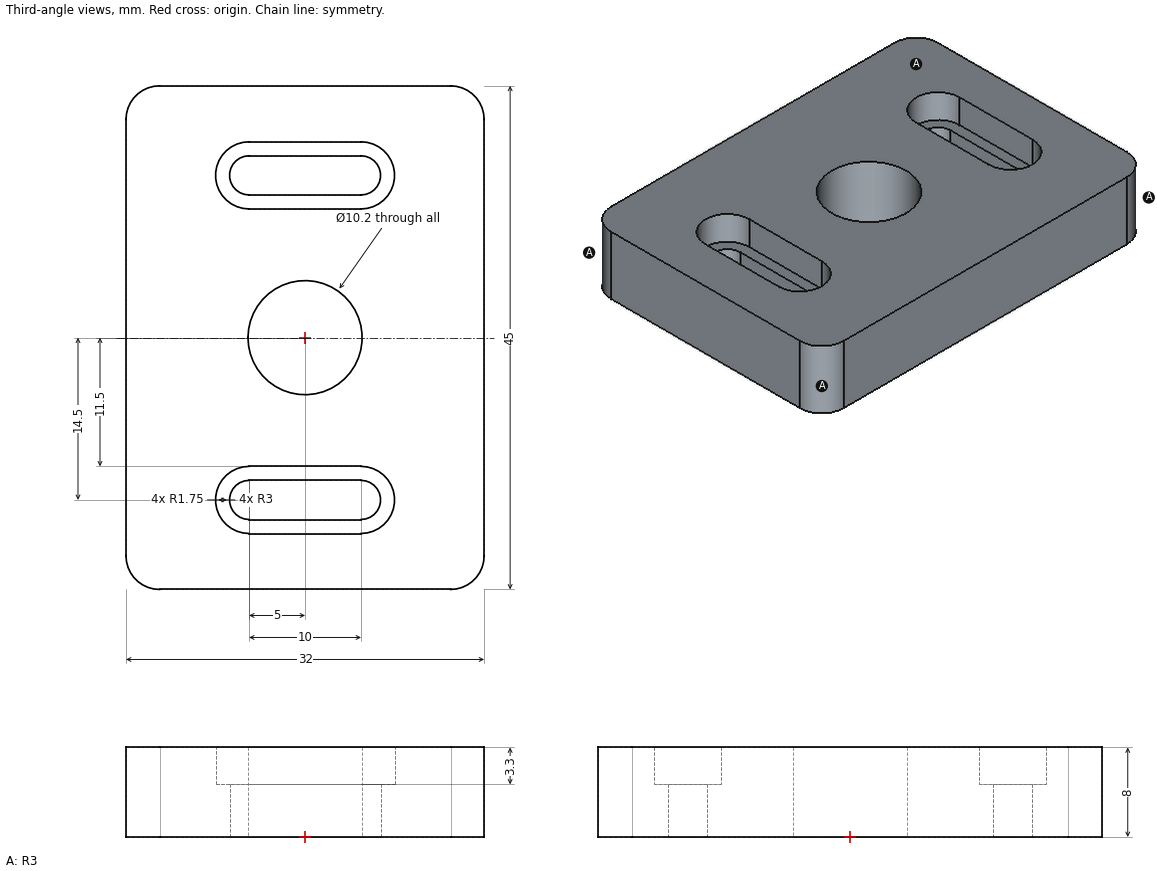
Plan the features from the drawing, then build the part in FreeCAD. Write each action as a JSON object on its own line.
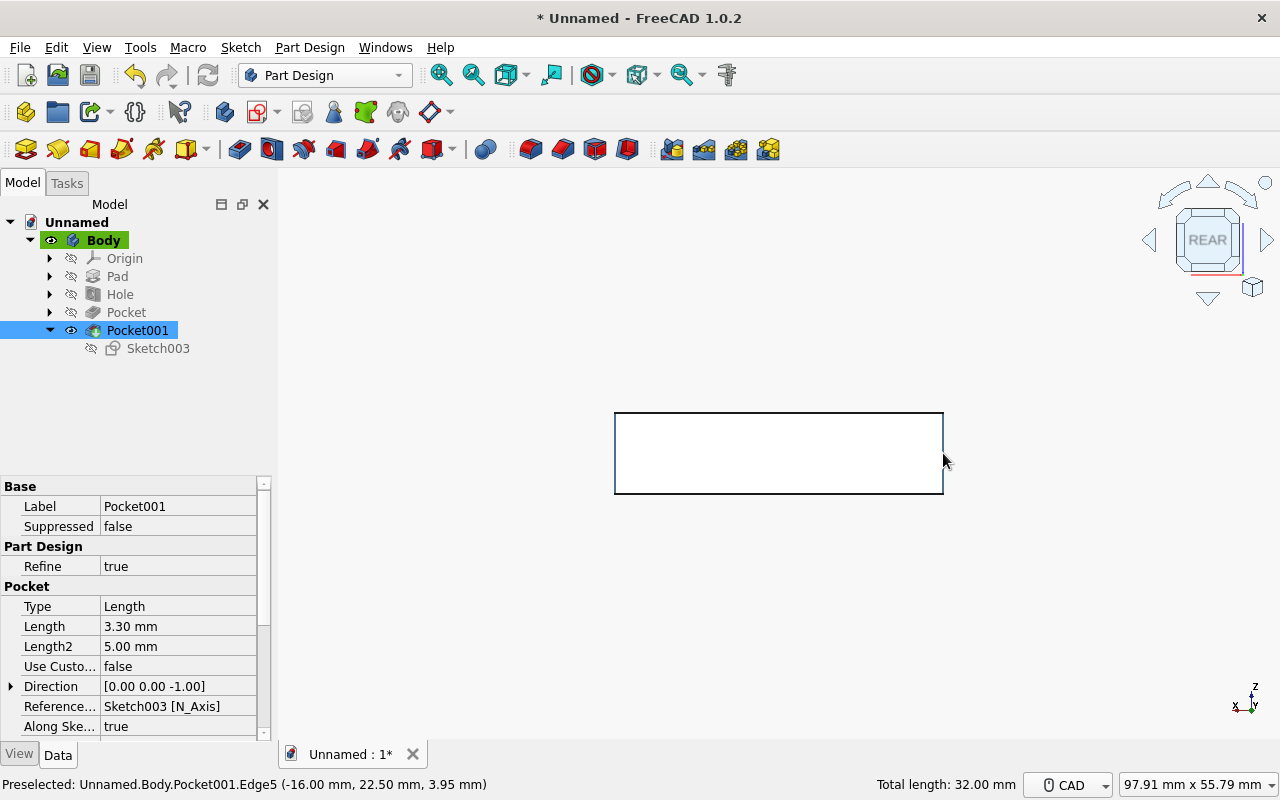
{"action": "left_click", "coordinate": [532, 150]}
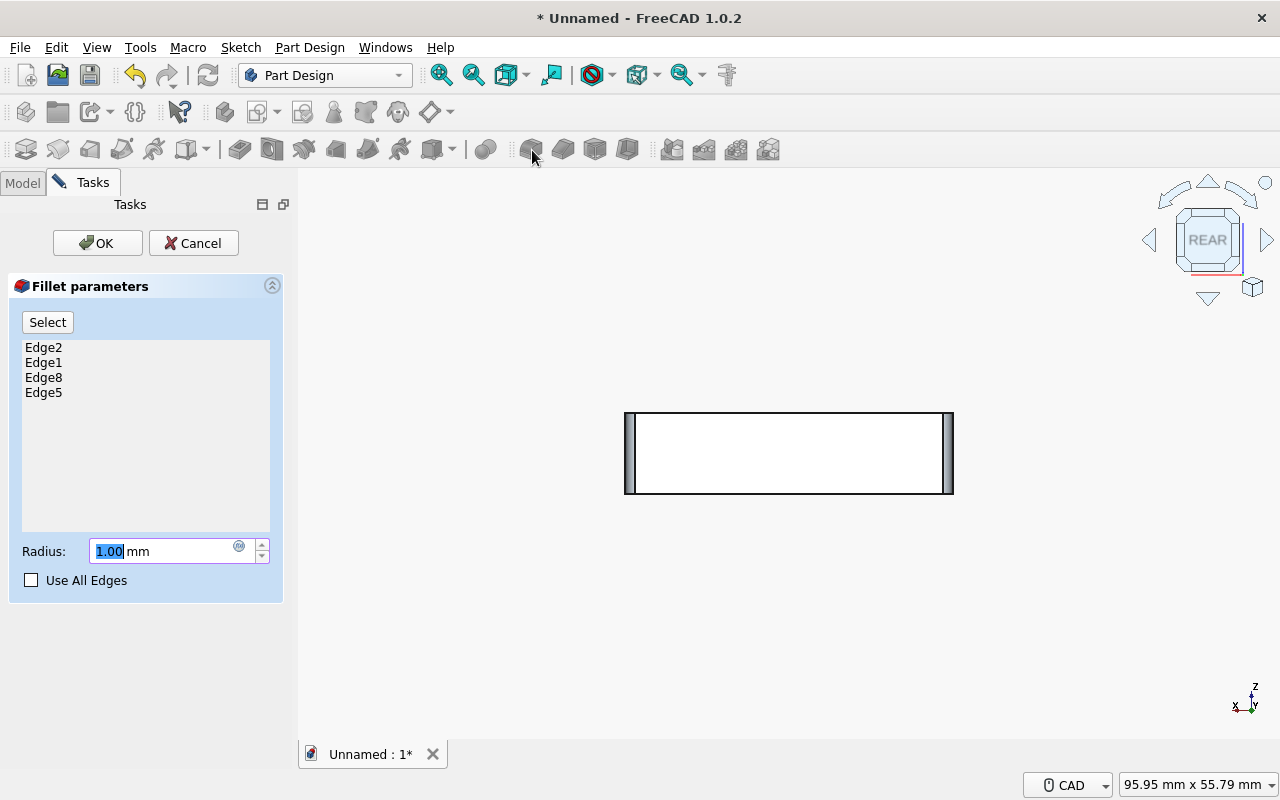
{"action": "type", "text": "3"}
{"action": "key", "text": "Tab"}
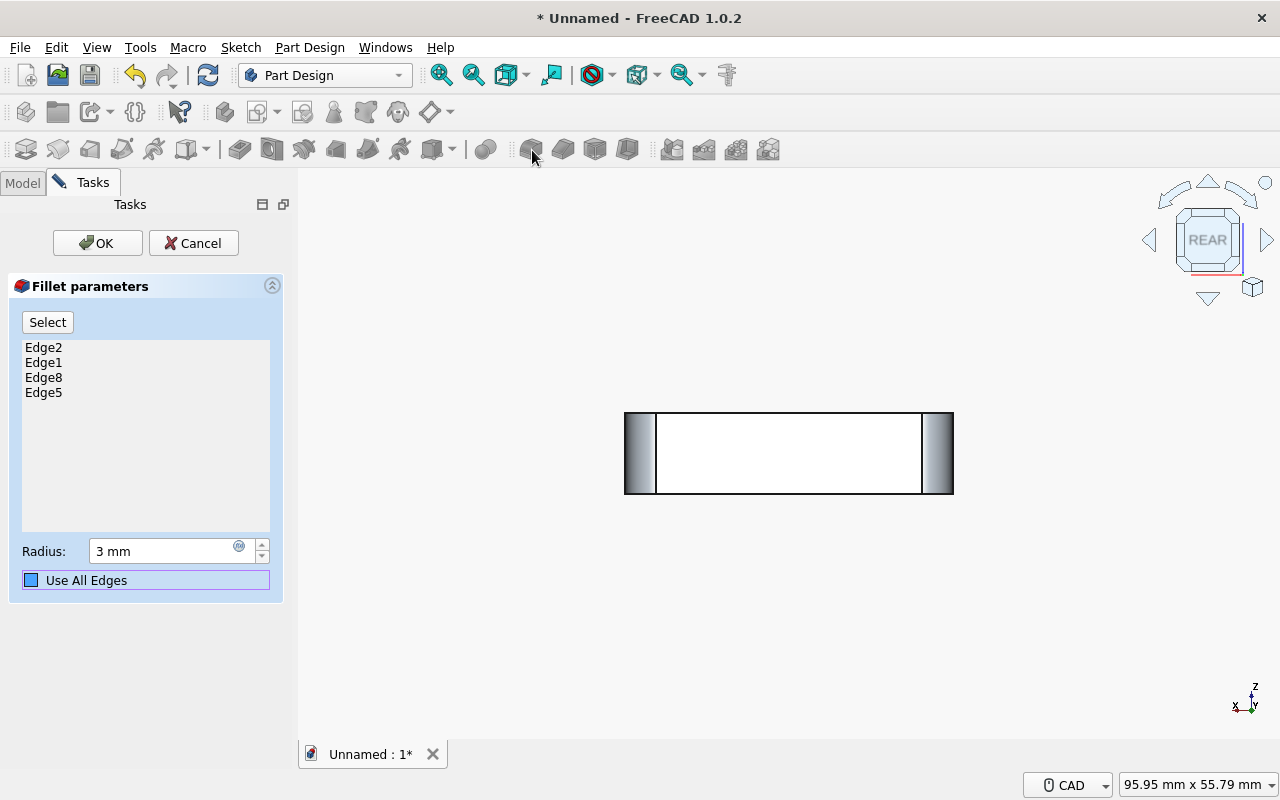
{"action": "left_click", "coordinate": [98, 243]}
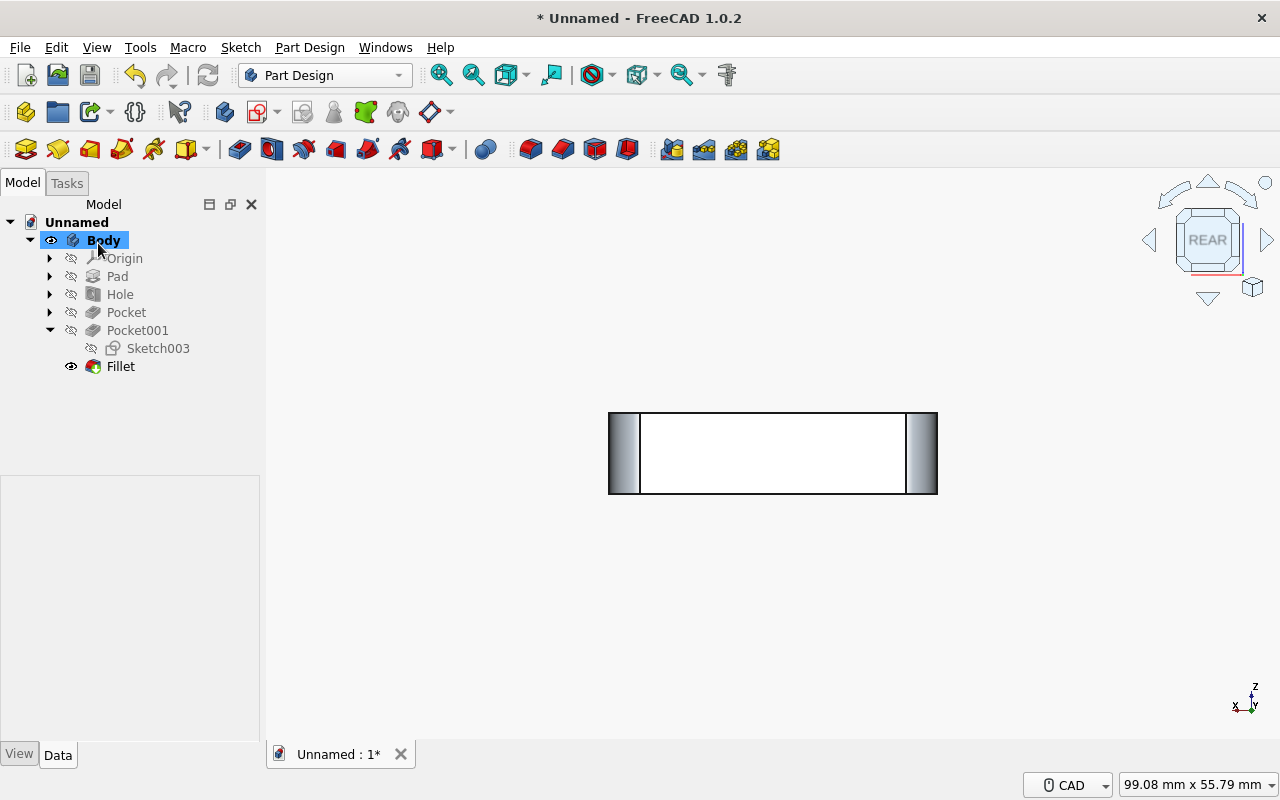
{"action": "key", "text": "0"}